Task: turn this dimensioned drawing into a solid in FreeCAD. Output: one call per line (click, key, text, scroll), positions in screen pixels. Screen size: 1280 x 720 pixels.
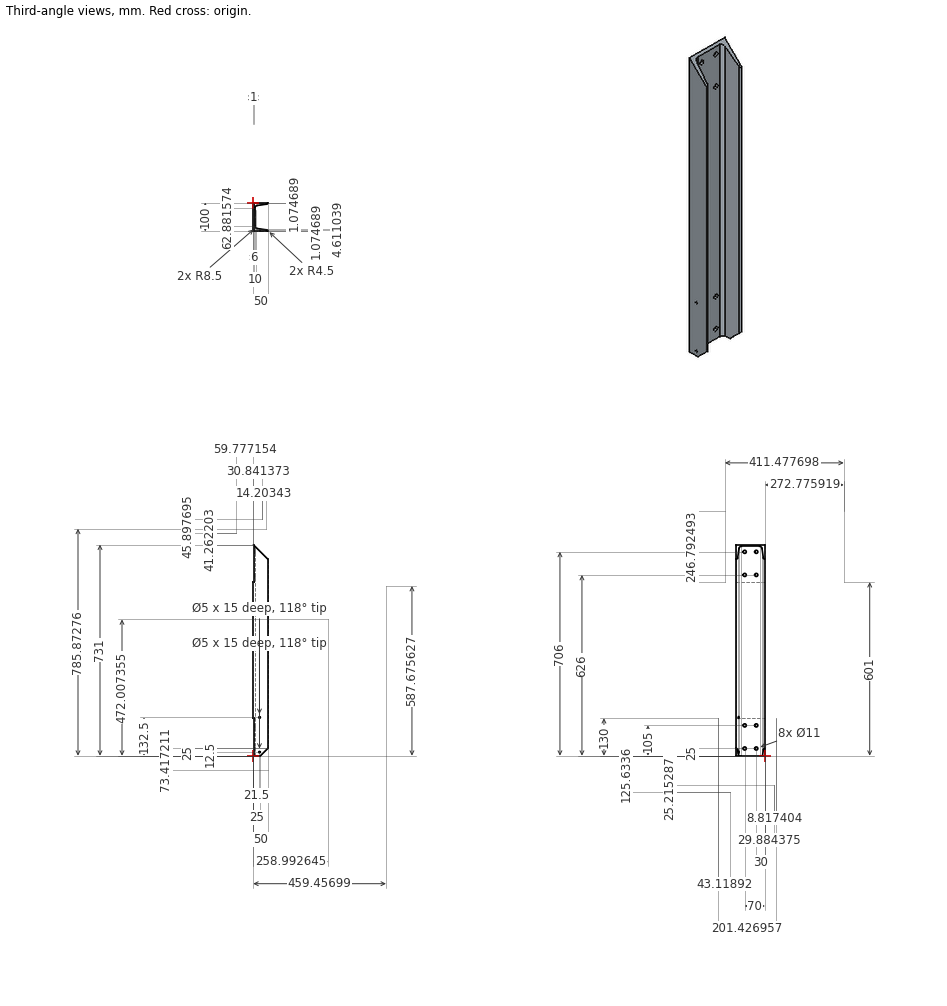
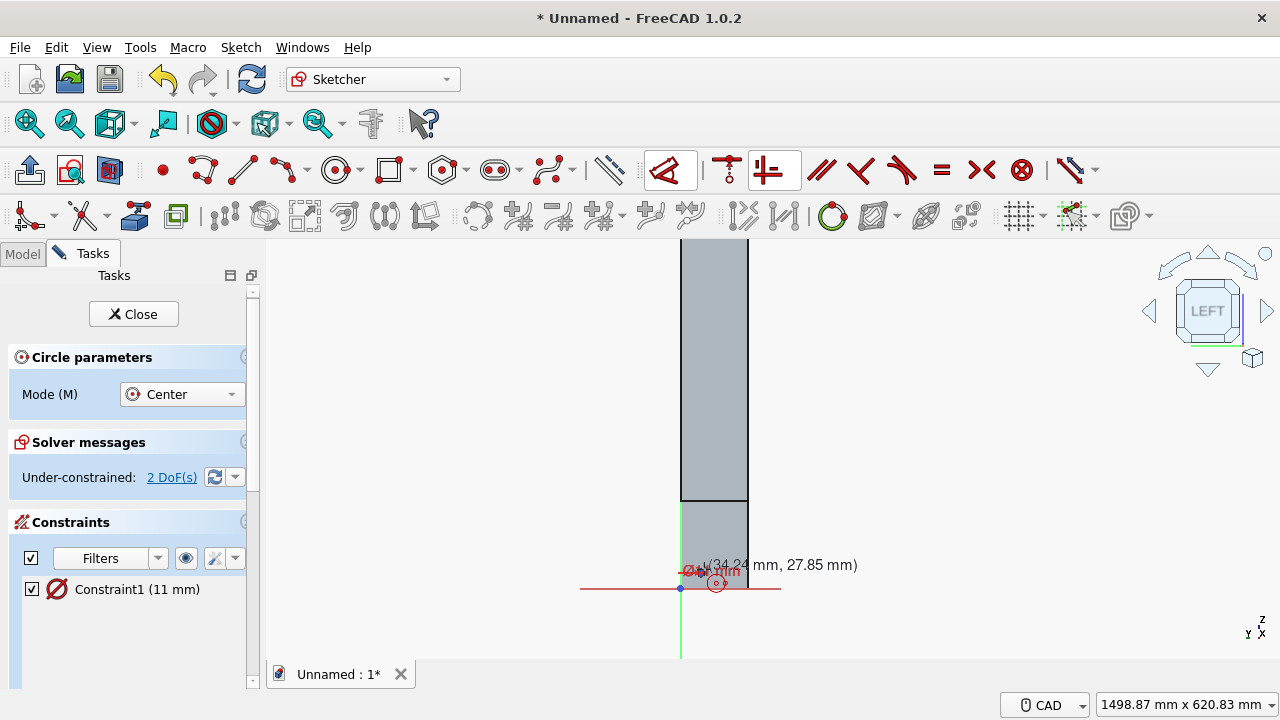
scroll(701, 518, up, 10)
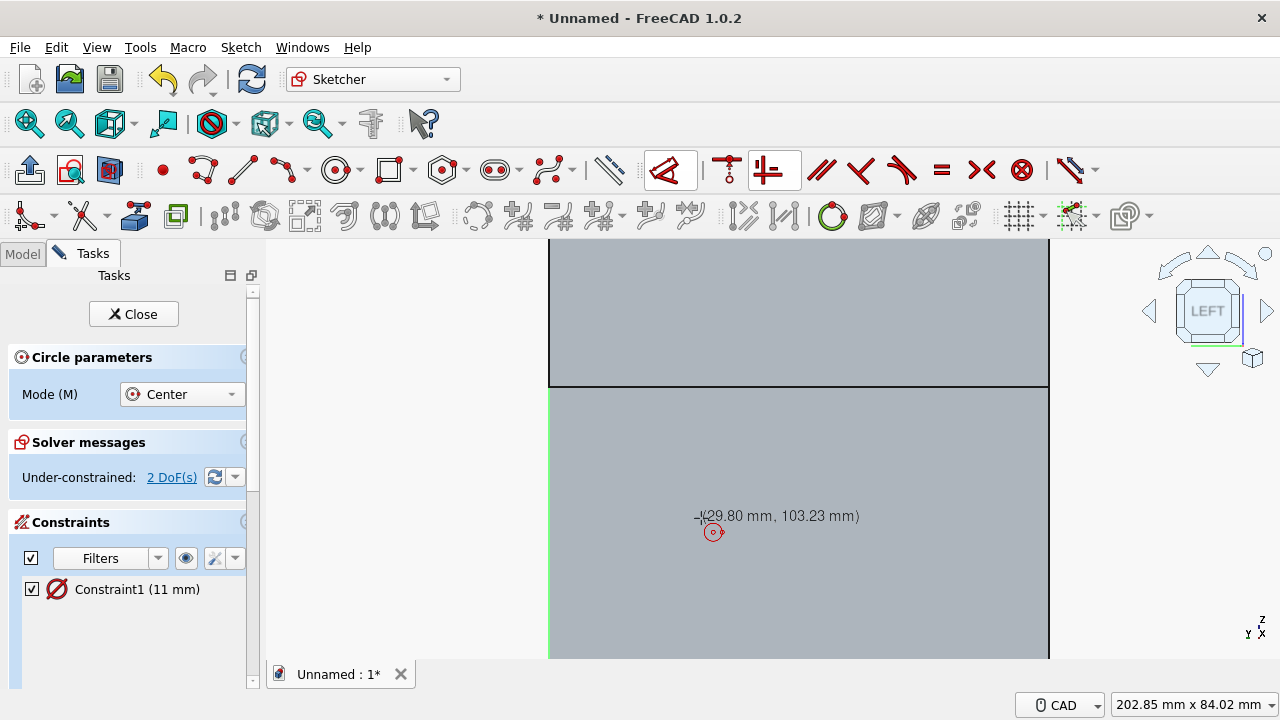
scroll(702, 544, down, 13)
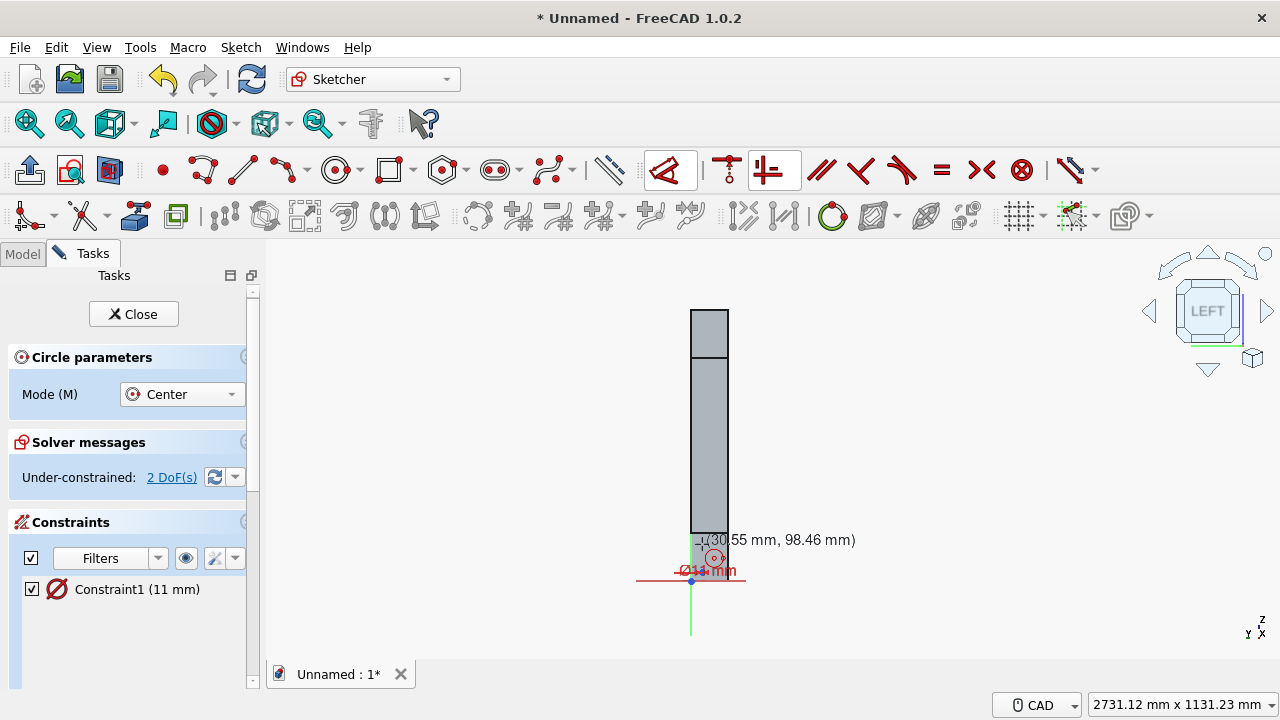
scroll(702, 542, up, 2)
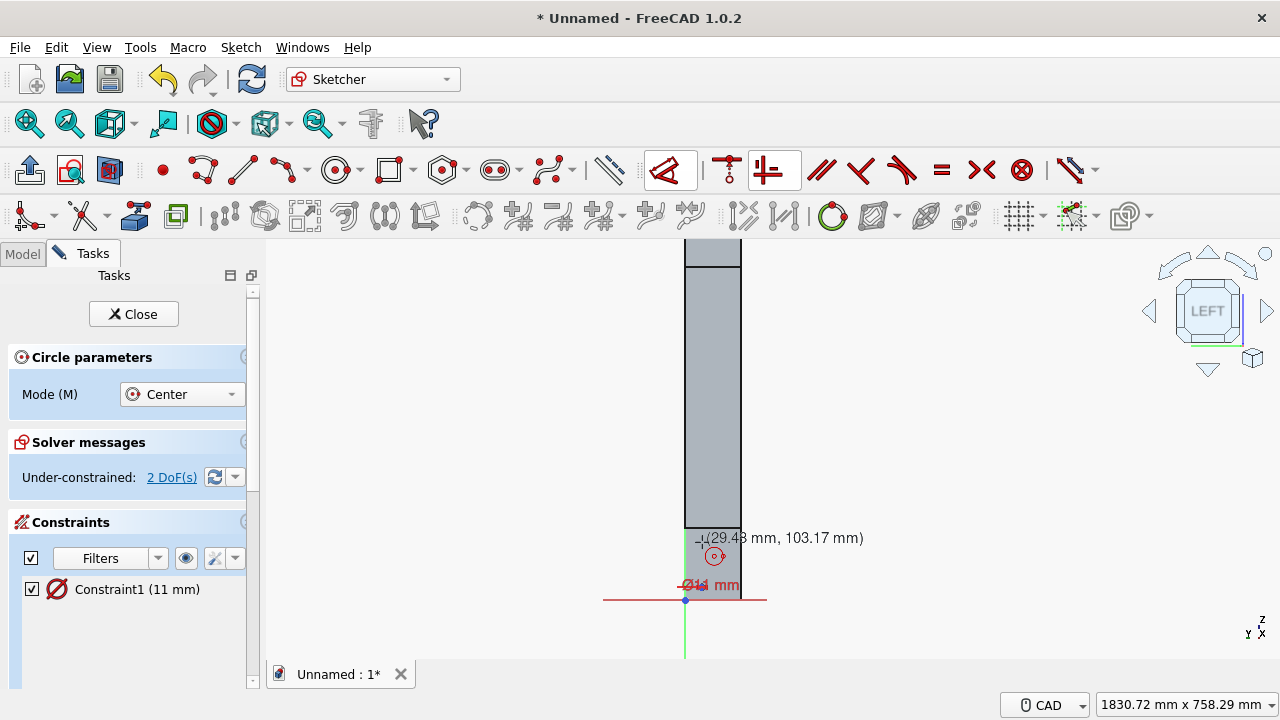
click(702, 542)
move(704, 540)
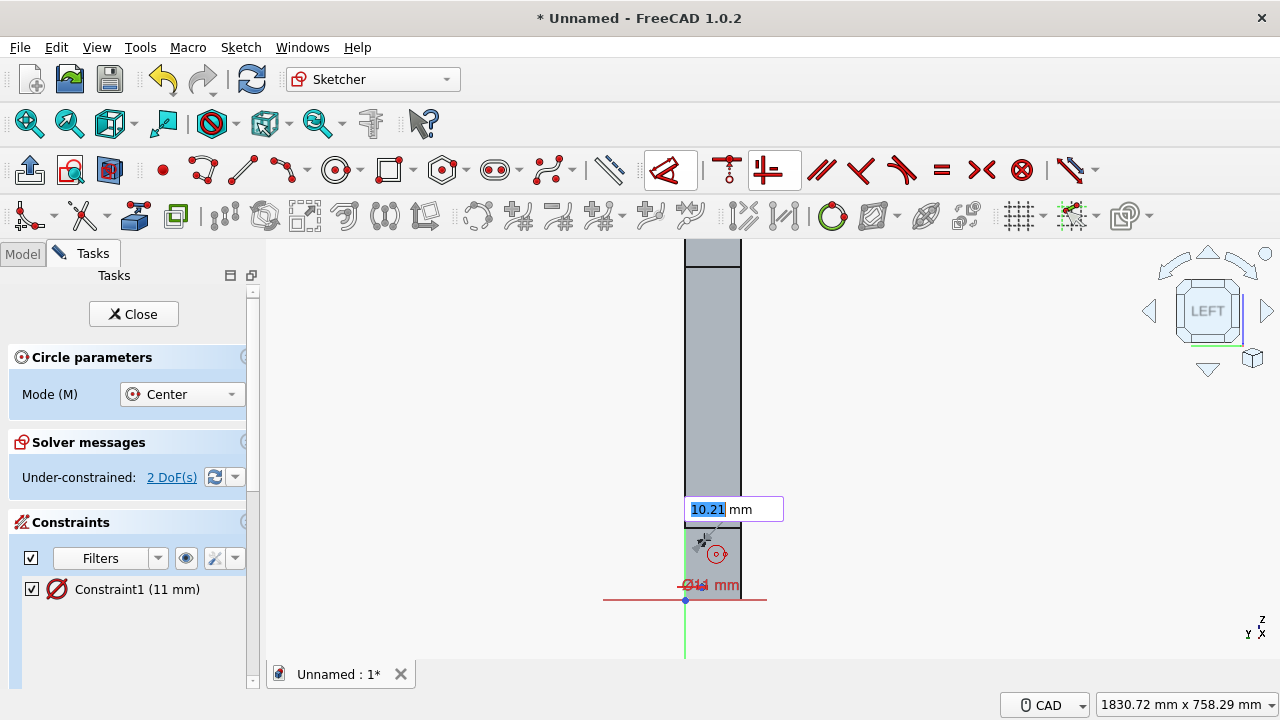
text(11)
key(Return)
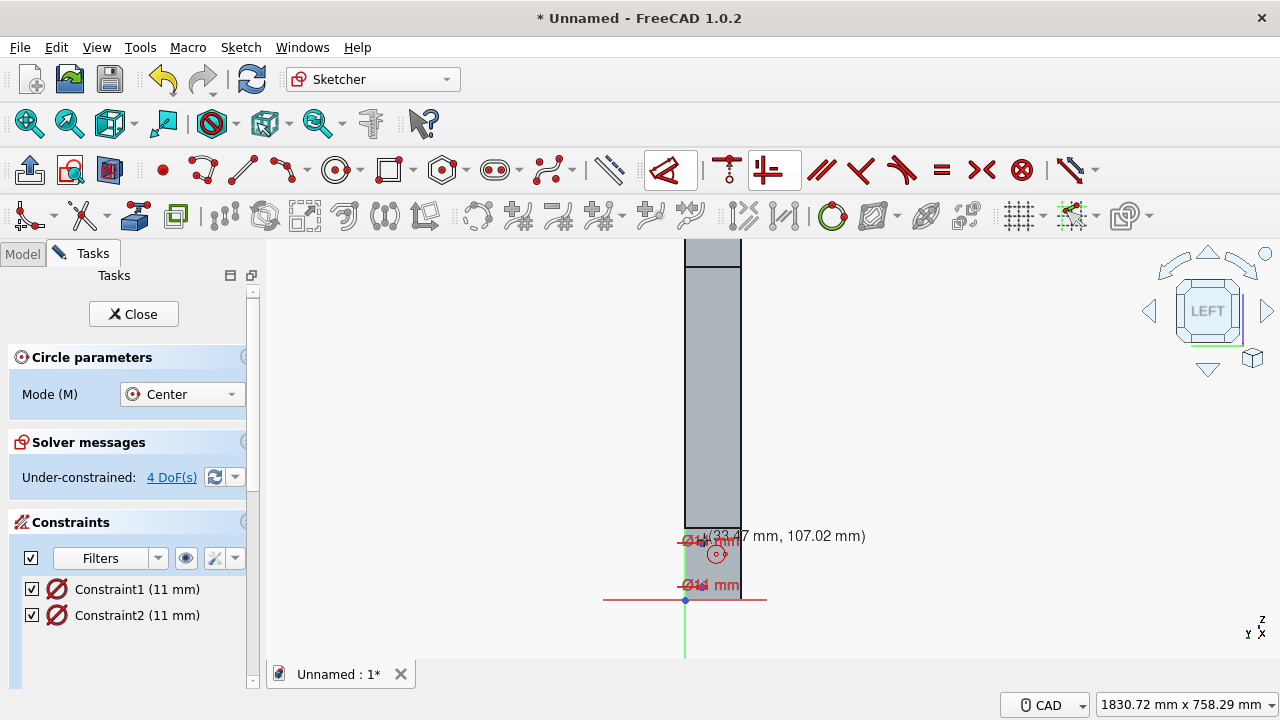
scroll(724, 586, up, 11)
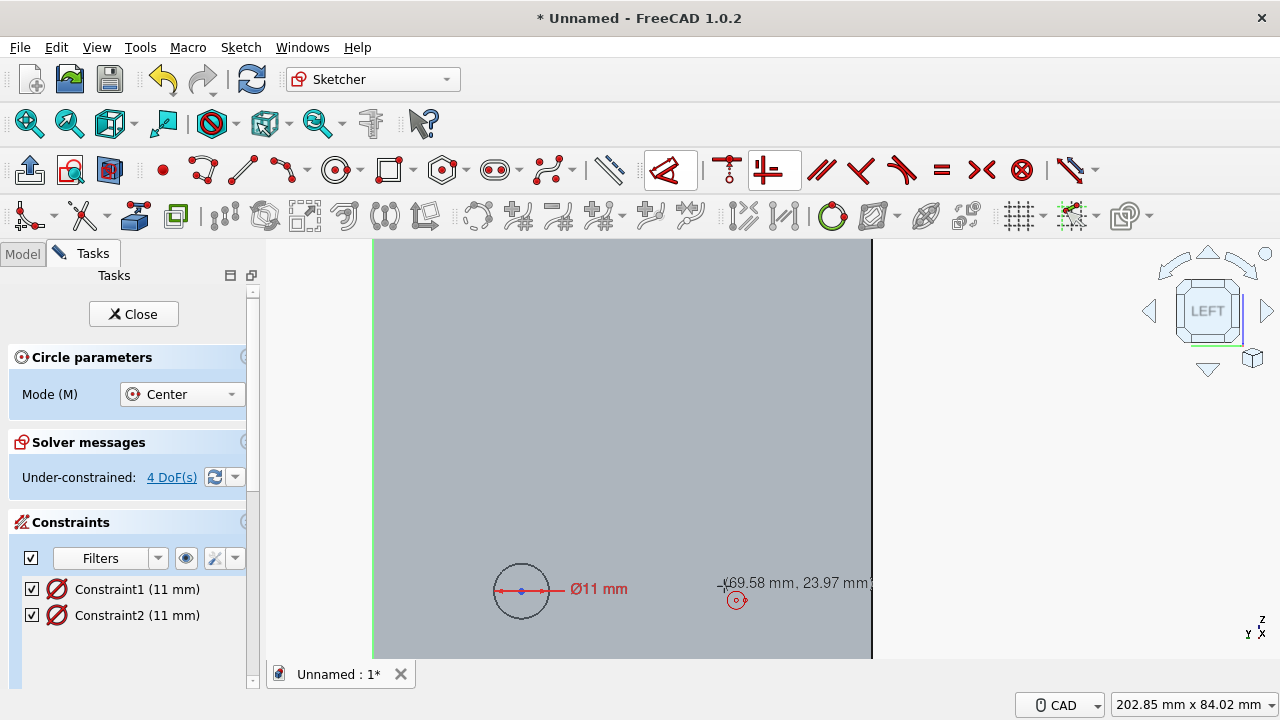
scroll(716, 571, down, 13)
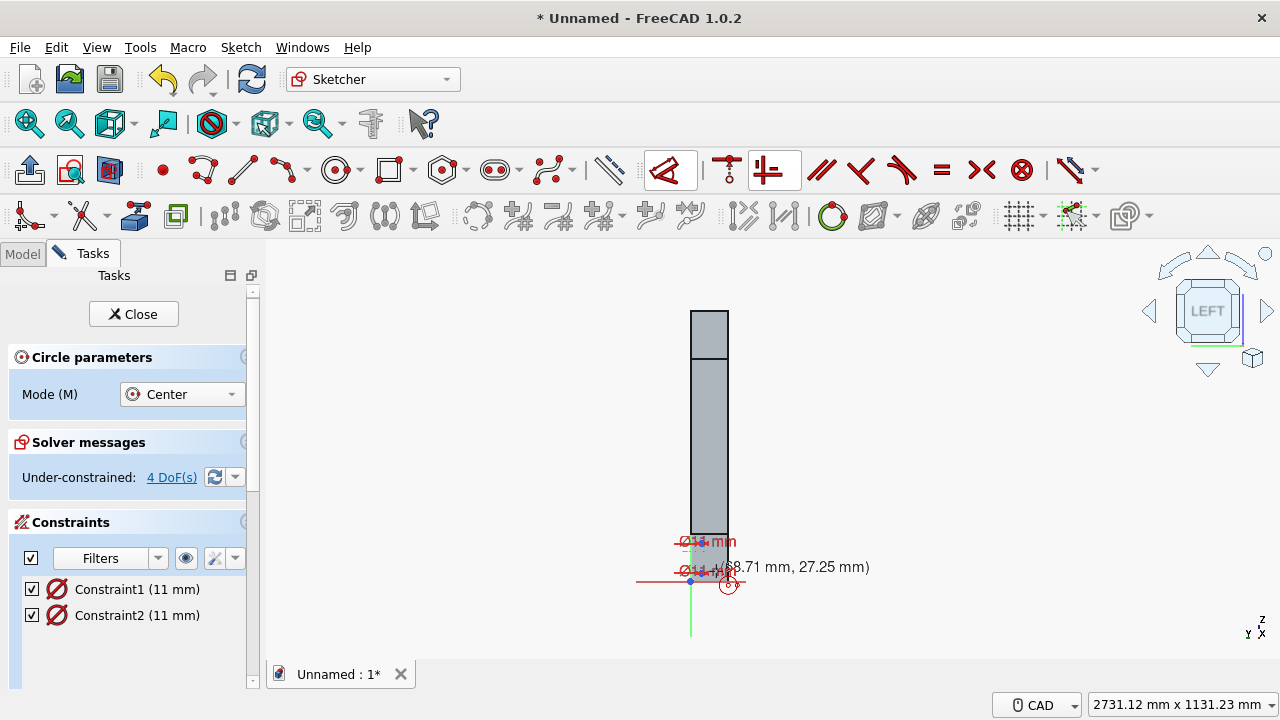
scroll(717, 573, up, 3)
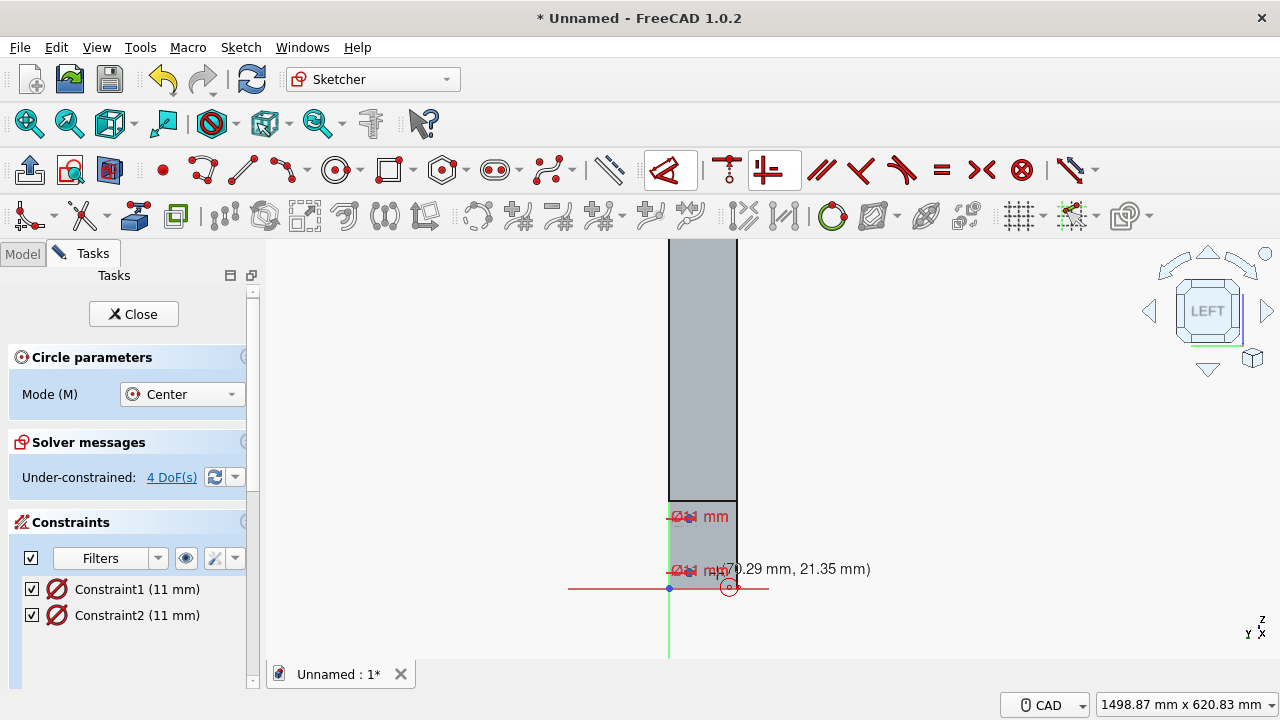
click(716, 572)
move(719, 569)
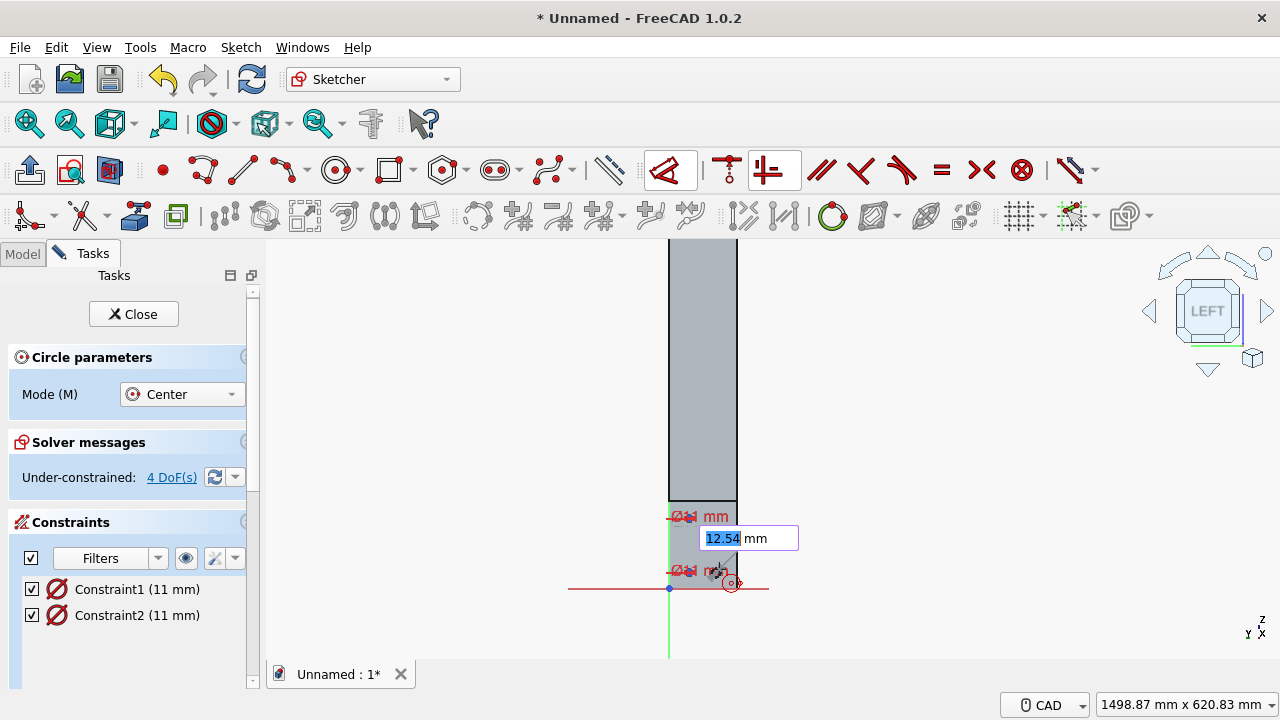
text(11)
key(Return)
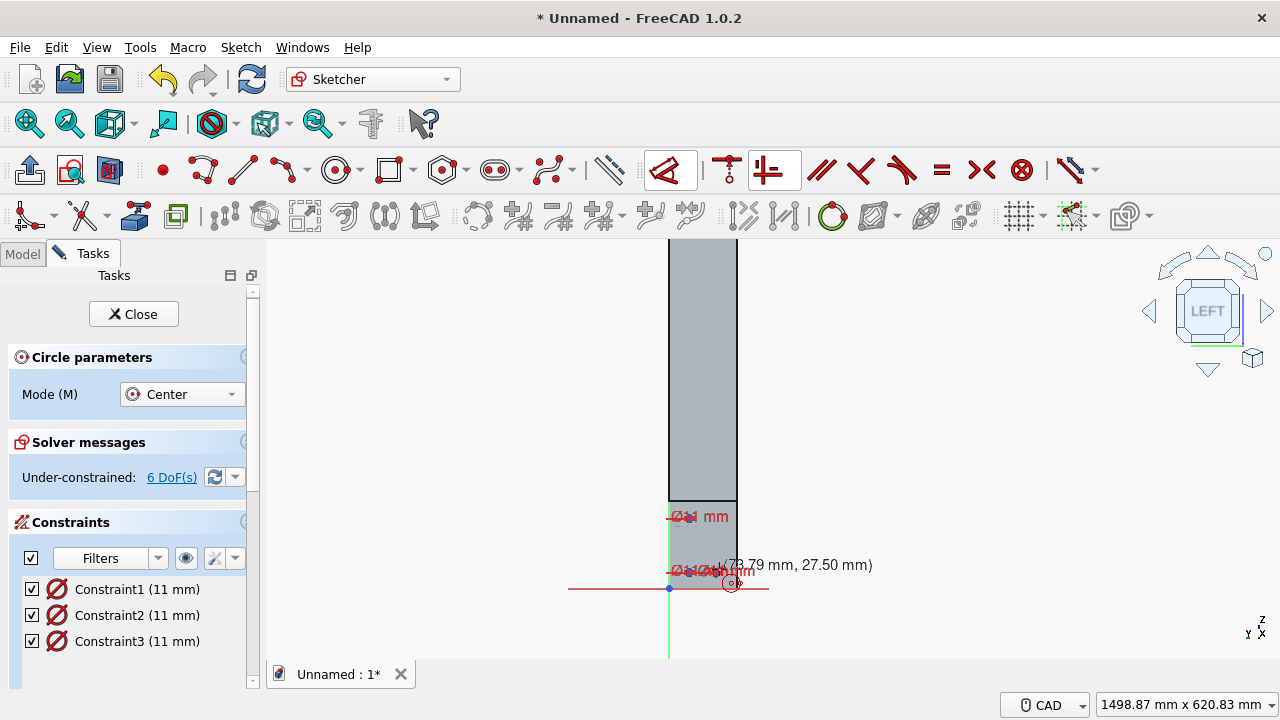
scroll(716, 518, up, 10)